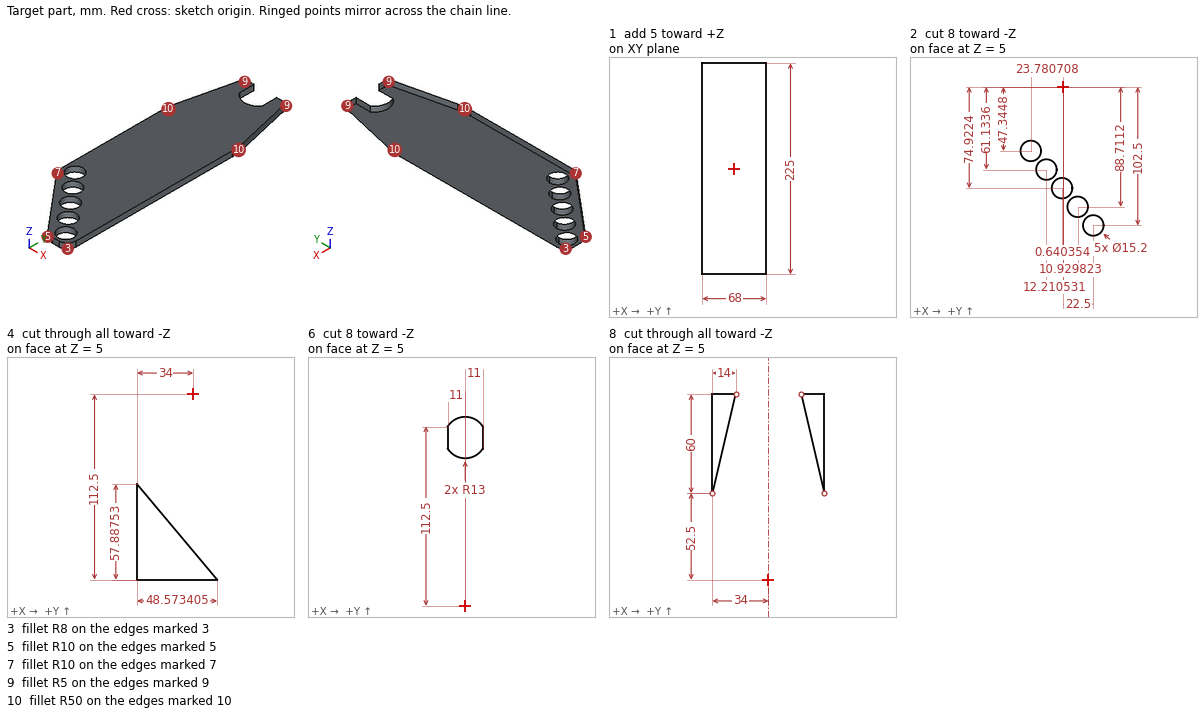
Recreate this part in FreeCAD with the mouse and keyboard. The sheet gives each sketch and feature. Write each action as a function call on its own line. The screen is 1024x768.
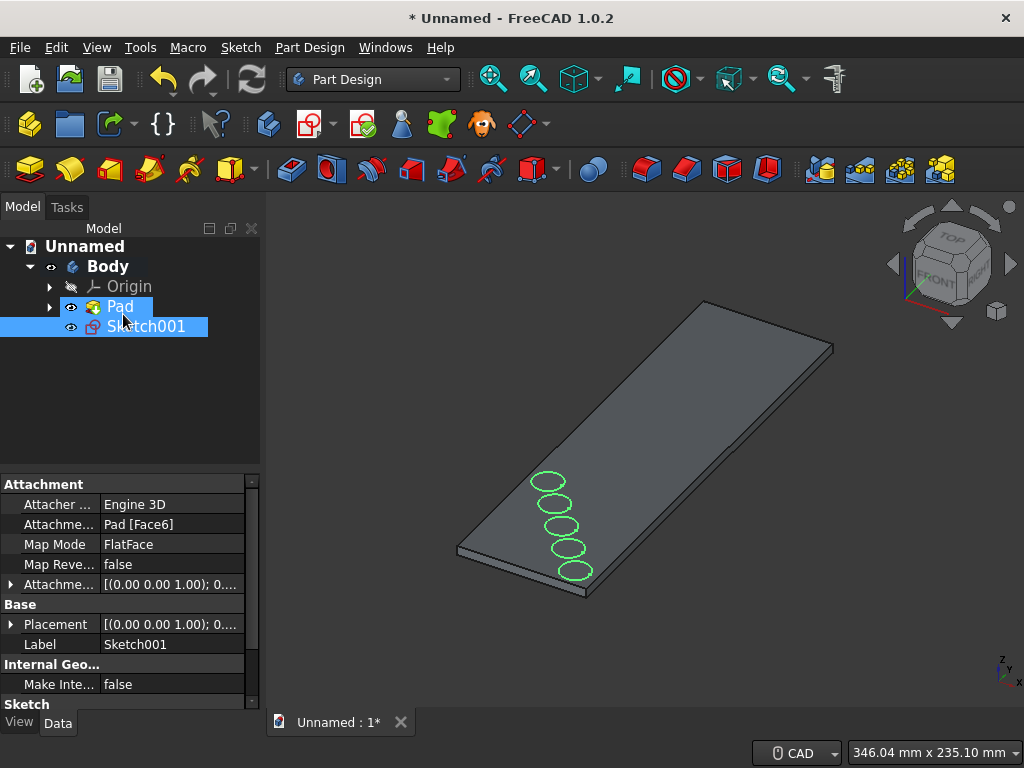
click(292, 170)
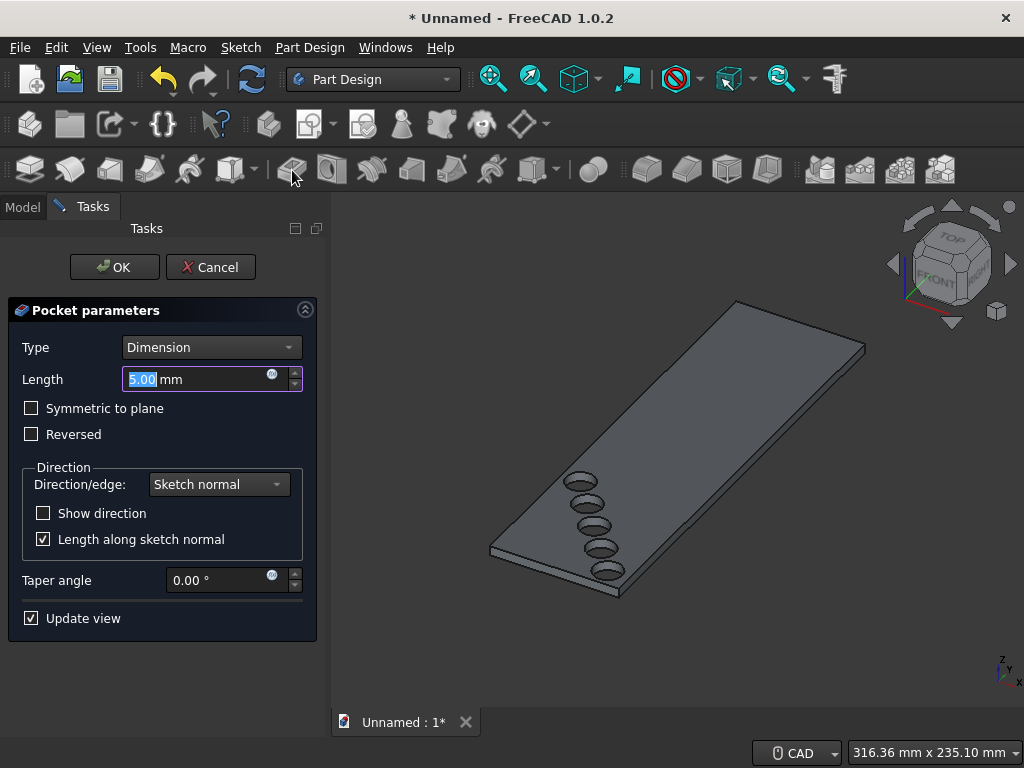
text(8)
key(Tab)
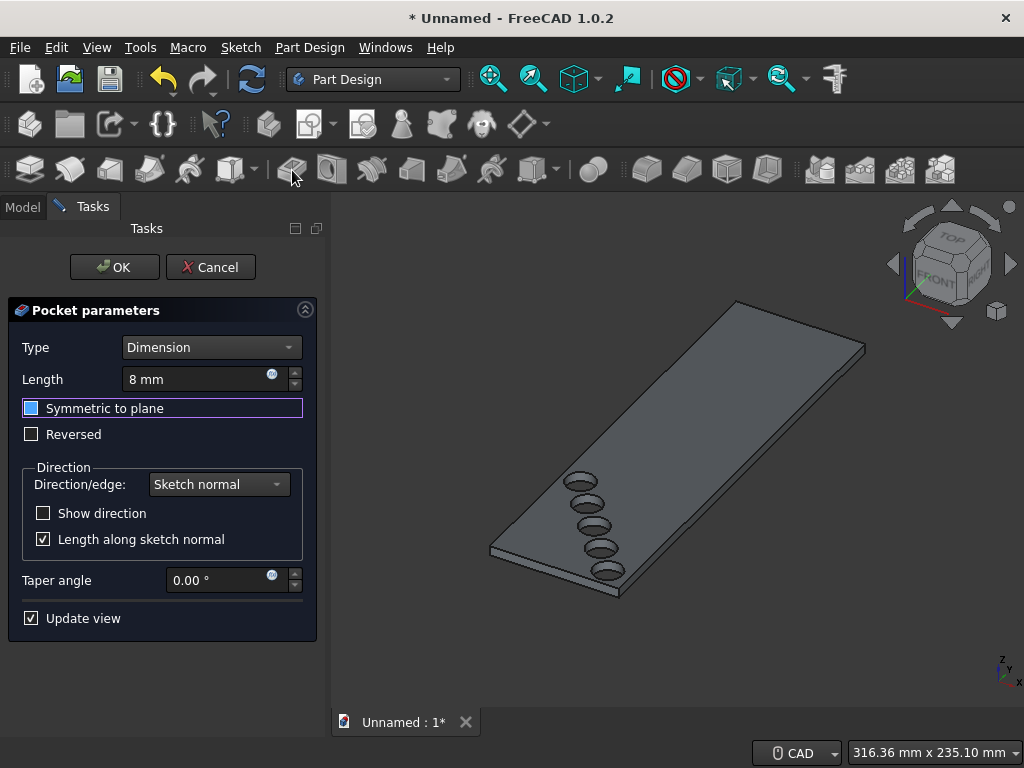
click(115, 267)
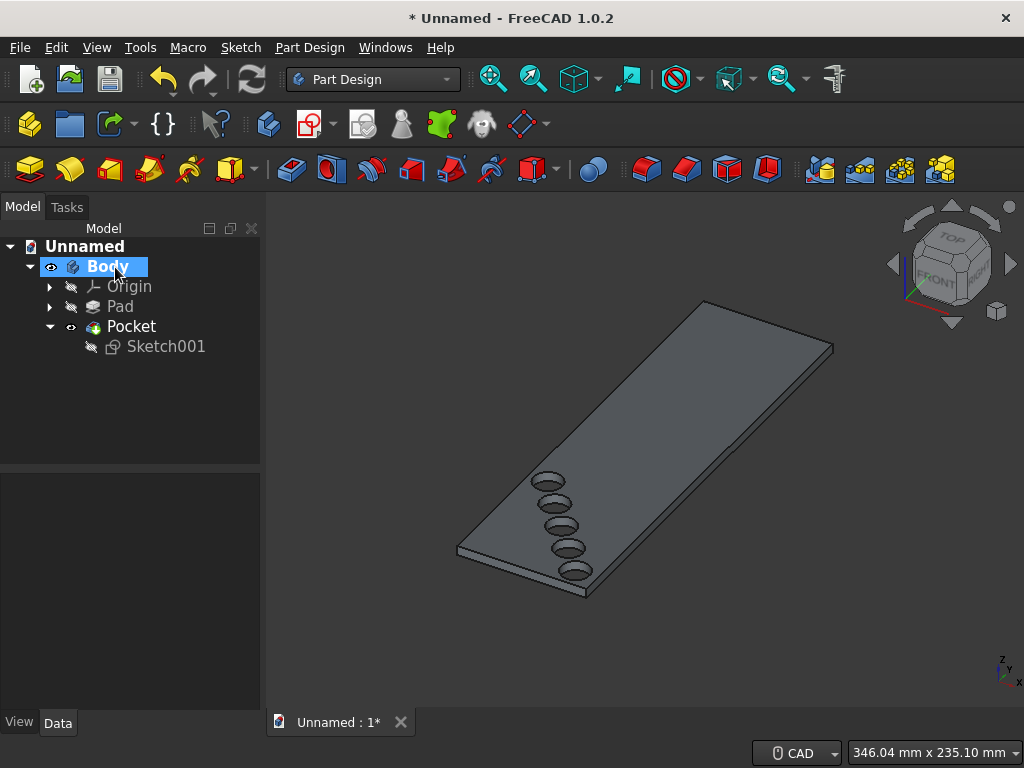
click(586, 594)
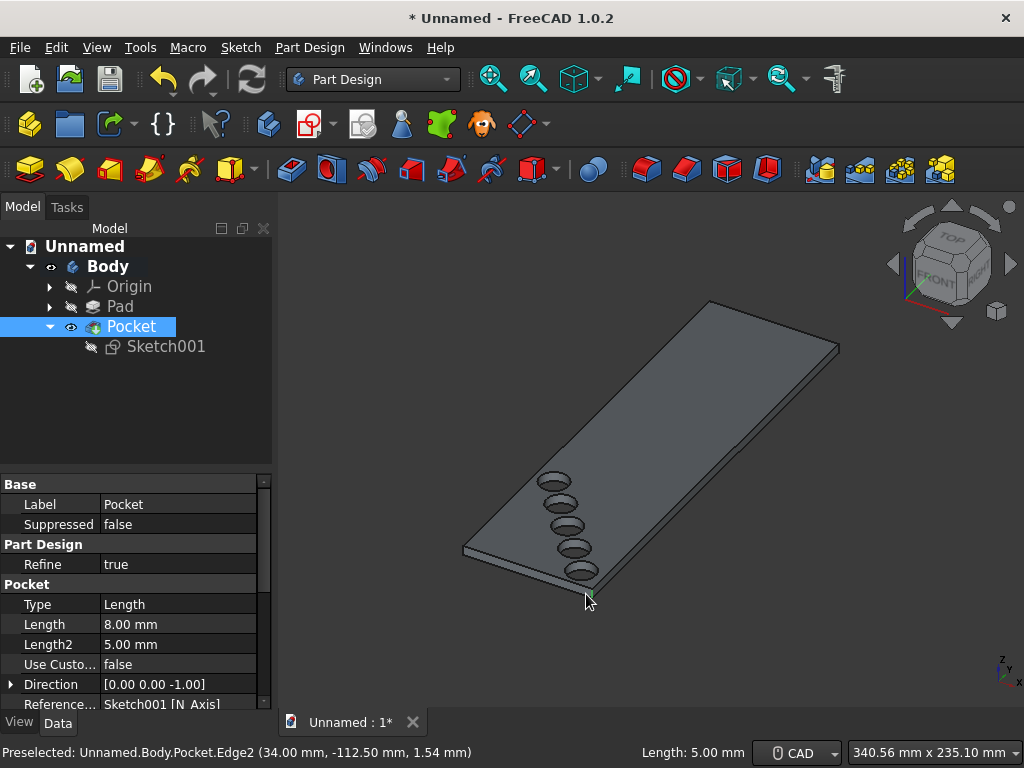
click(648, 170)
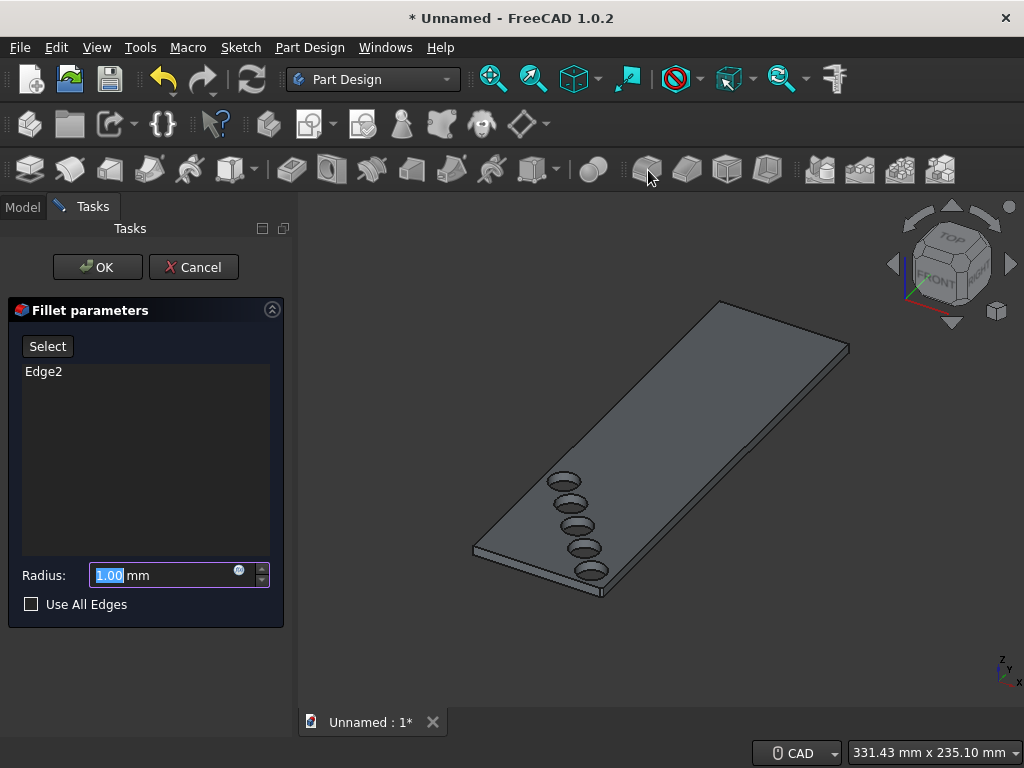
text(8)
key(Tab)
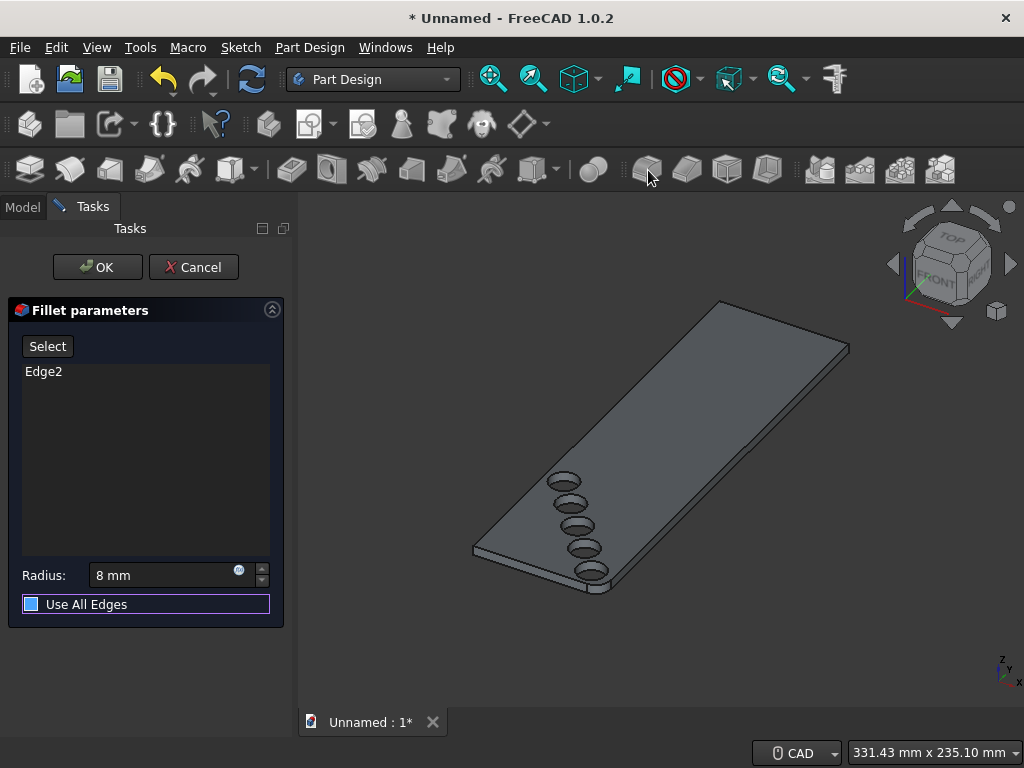
click(98, 267)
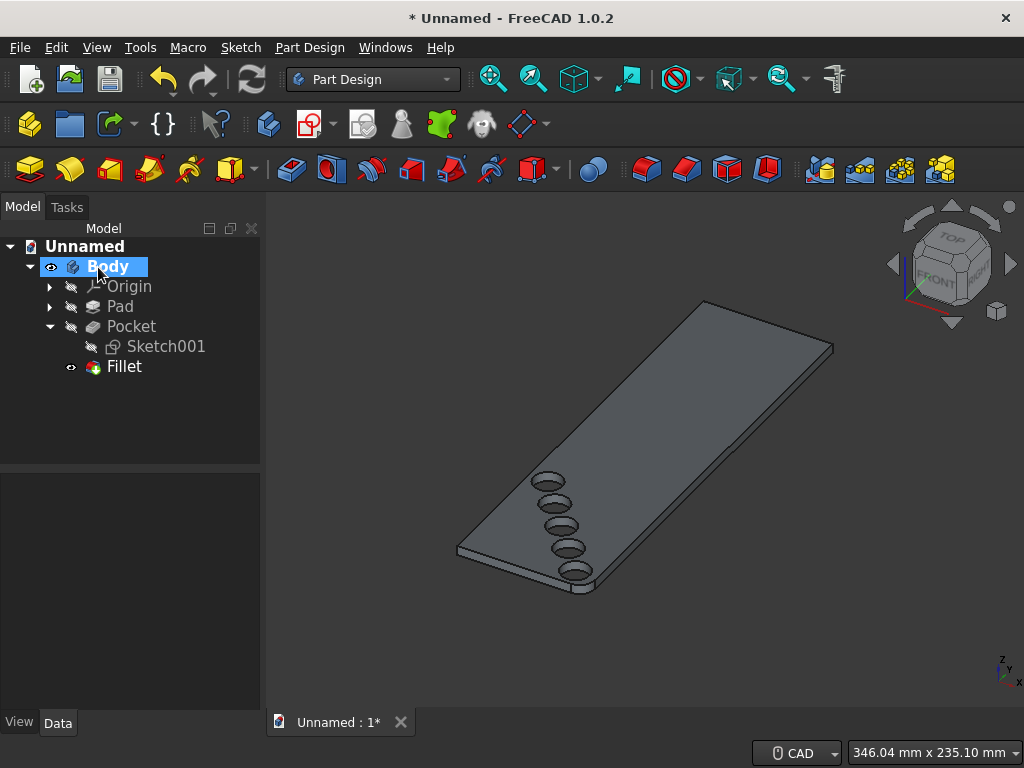
click(715, 374)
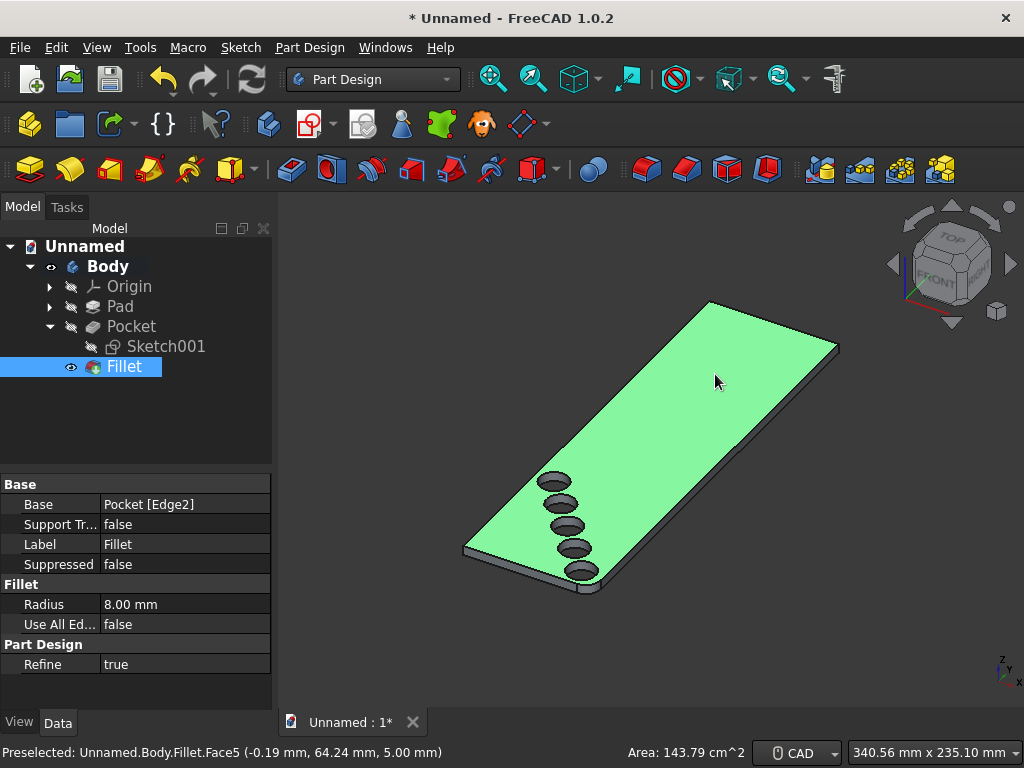
click(310, 124)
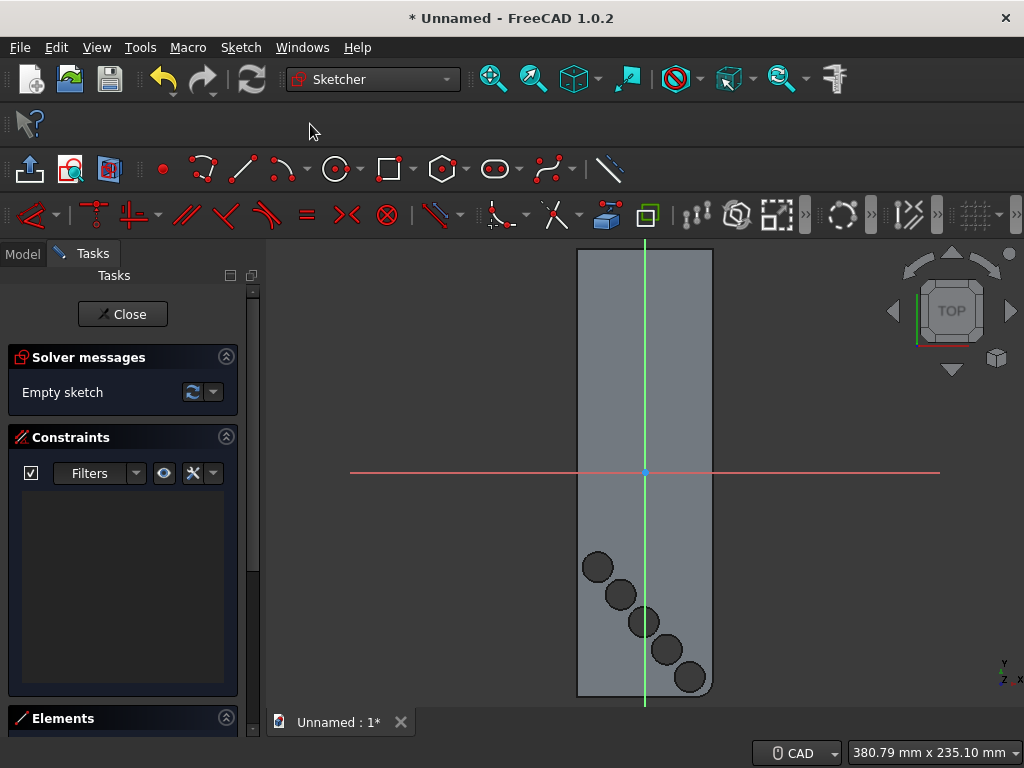
scroll(354, 267, down, 1)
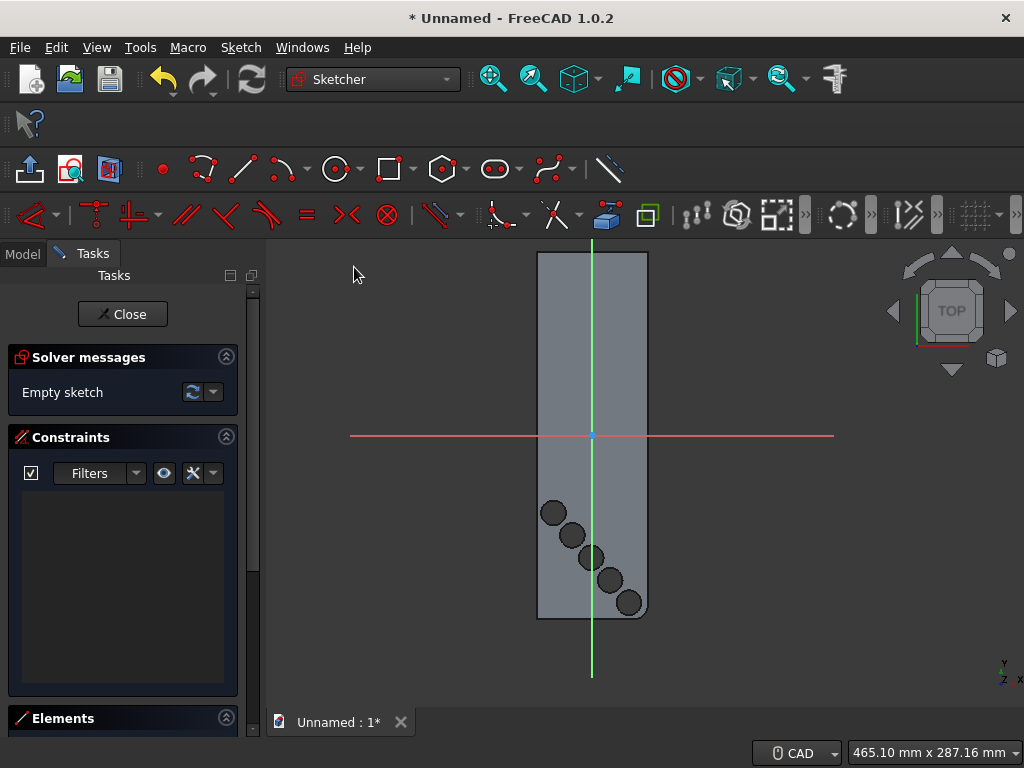
scroll(576, 638, up, 2)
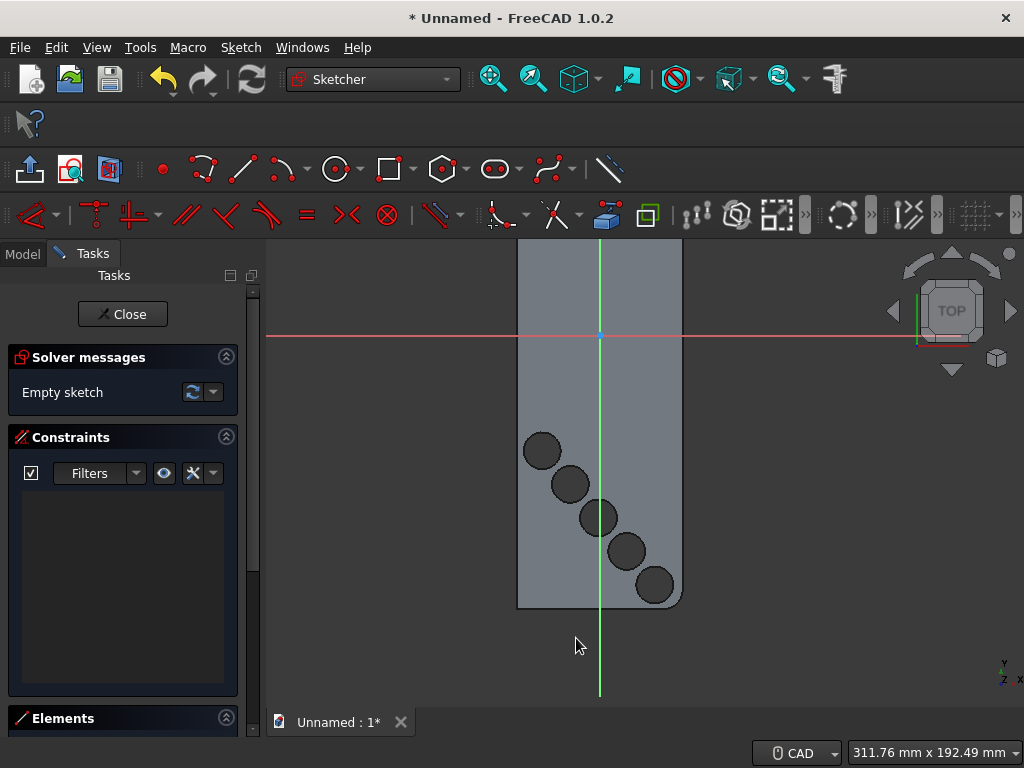
key(g)
key(m)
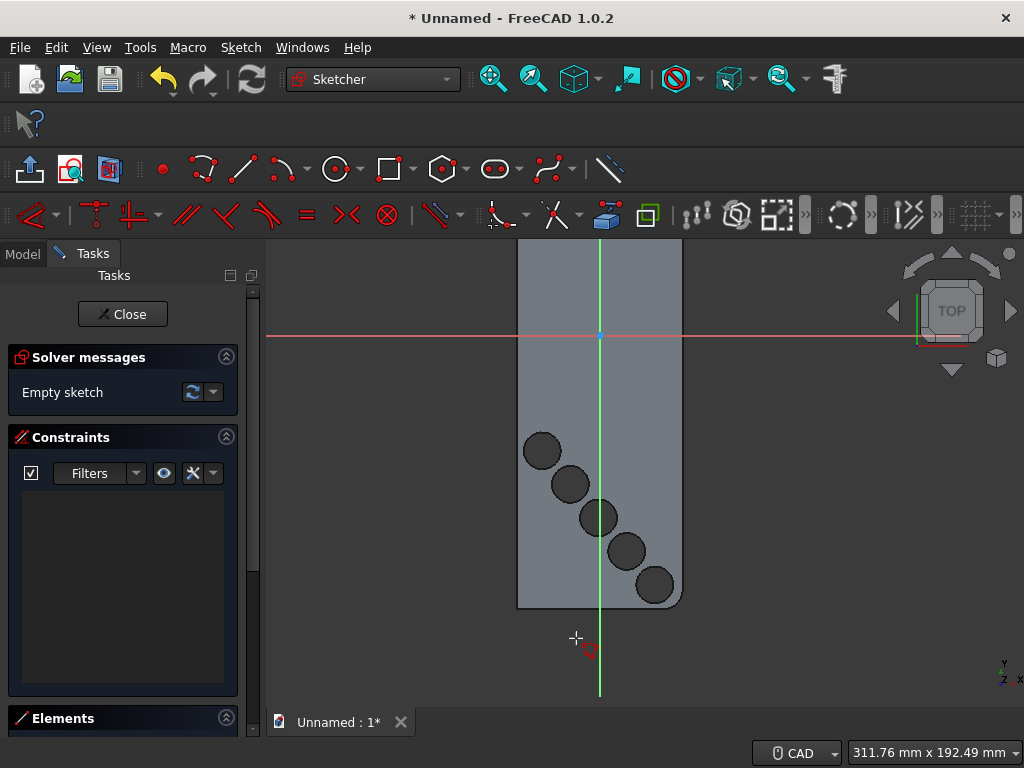
click(517, 469)
click(517, 609)
click(636, 609)
click(517, 470)
key(Escape)
key(Escape)